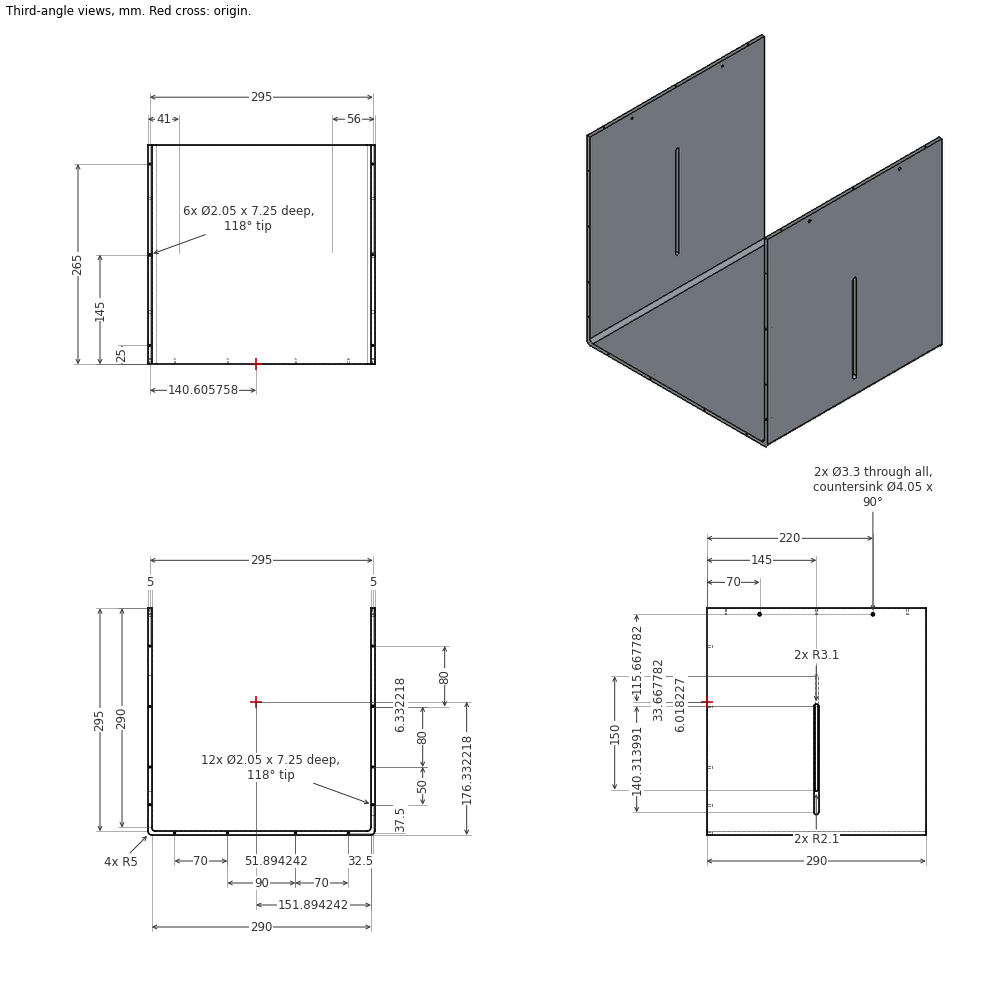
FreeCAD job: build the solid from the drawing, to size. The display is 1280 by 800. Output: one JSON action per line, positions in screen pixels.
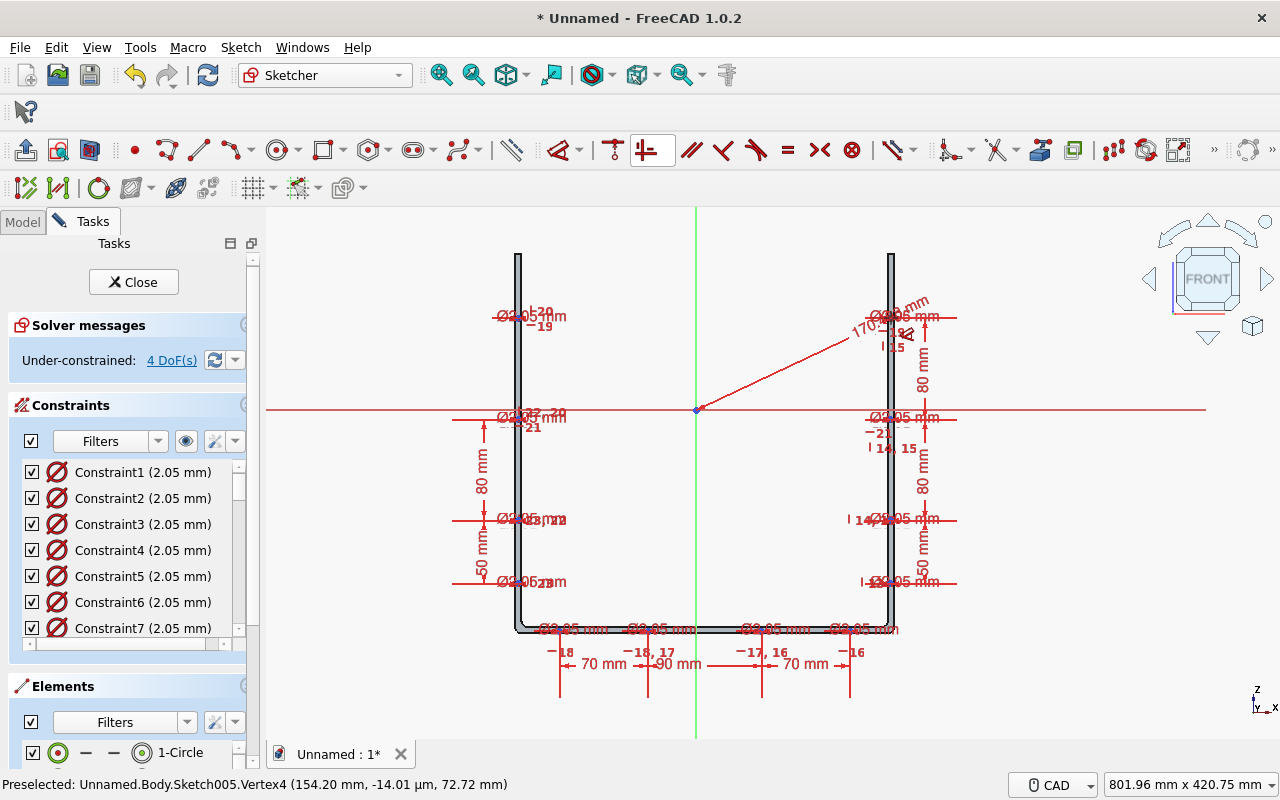
{"action": "left_click", "coordinate": [518, 318]}
{"action": "left_click", "coordinate": [619, 284]}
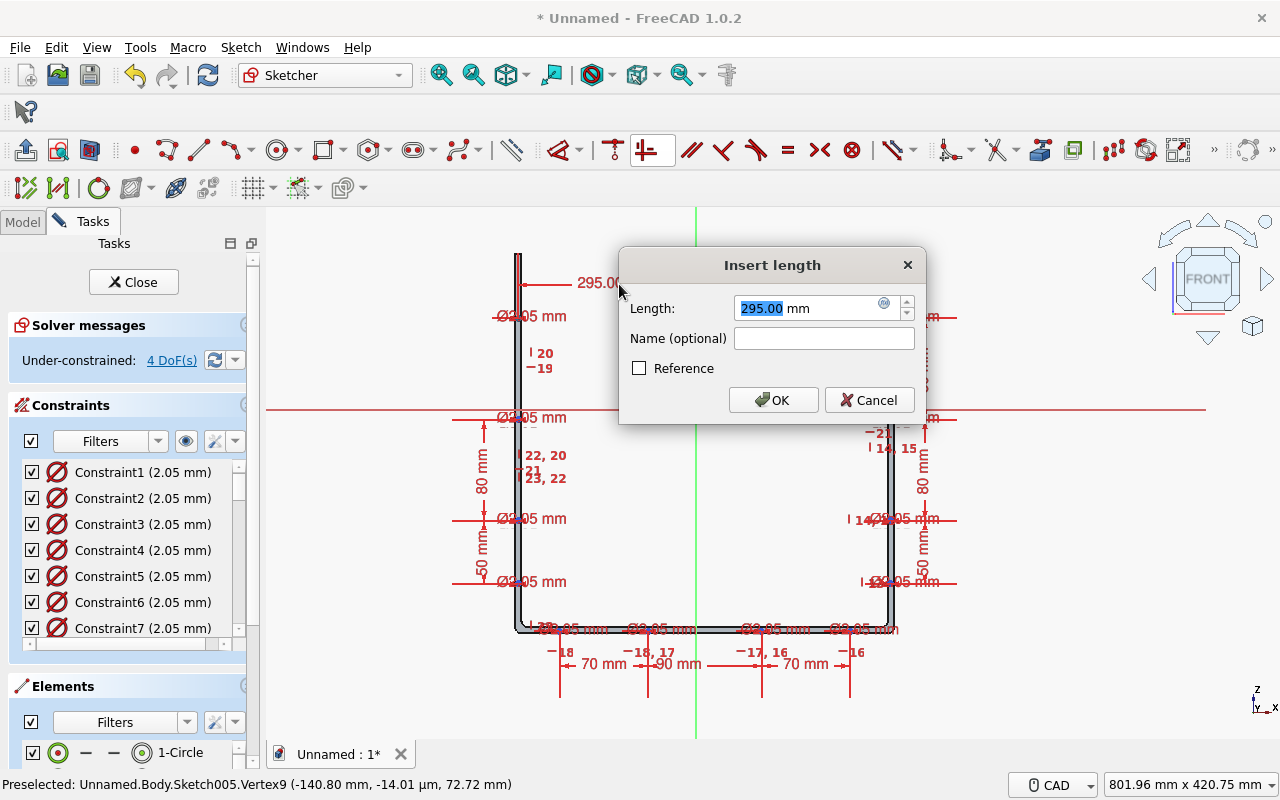
{"action": "type", "text": "295"}
{"action": "key", "text": "Return"}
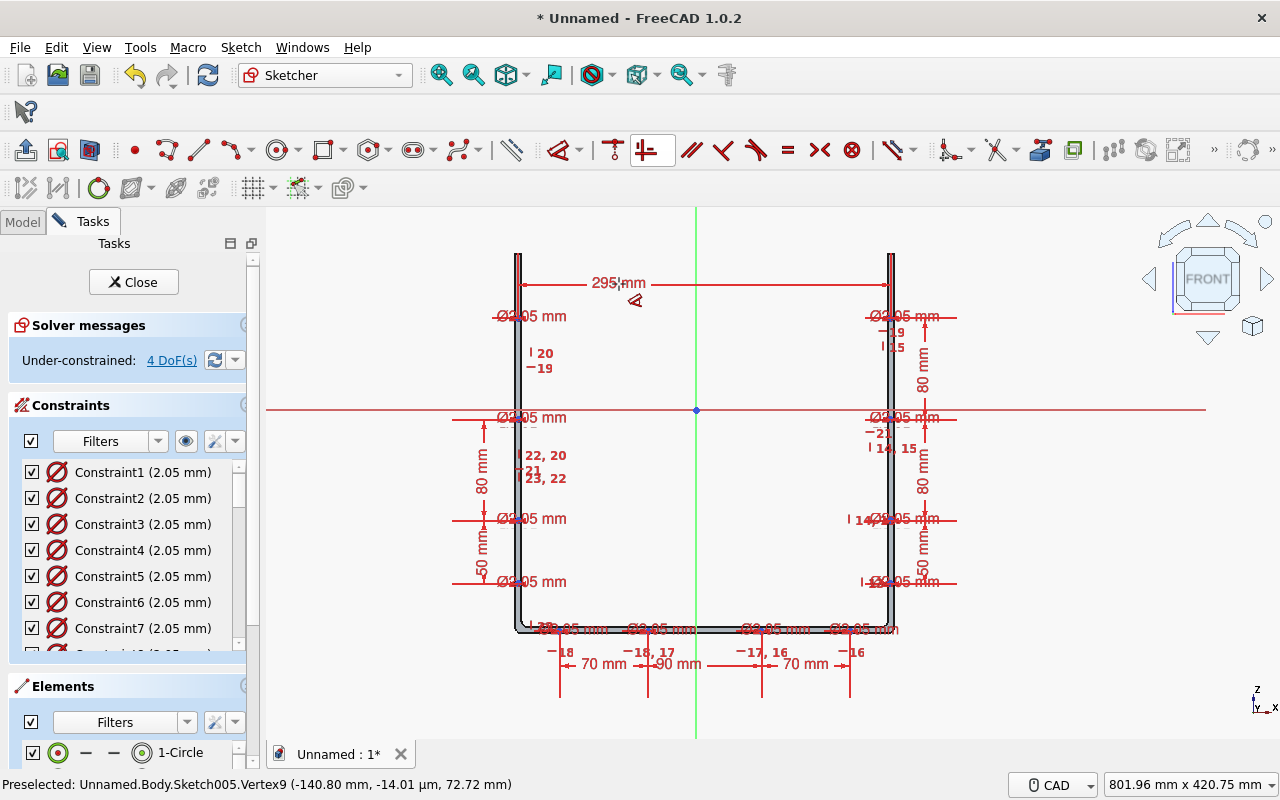
{"action": "left_click", "coordinate": [891, 584]}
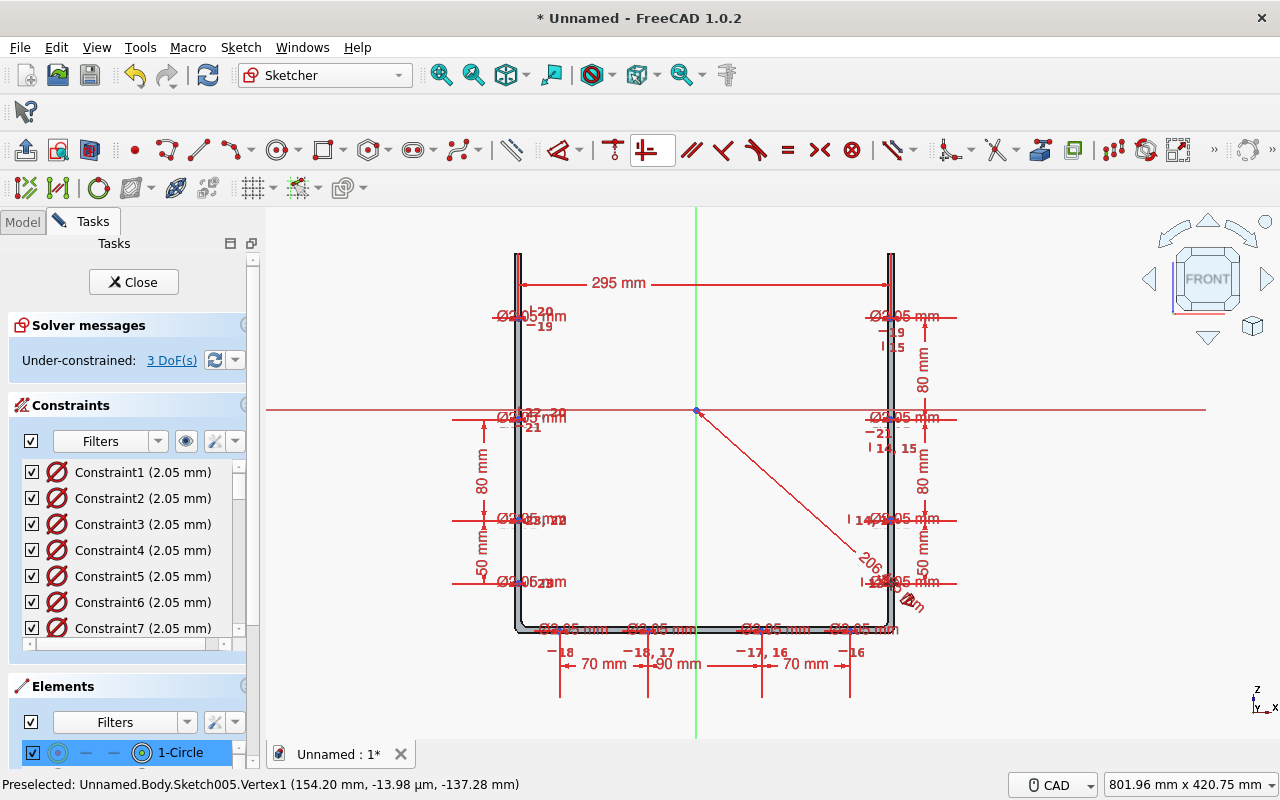
{"action": "left_click", "coordinate": [850, 631]}
{"action": "left_click", "coordinate": [880, 665]}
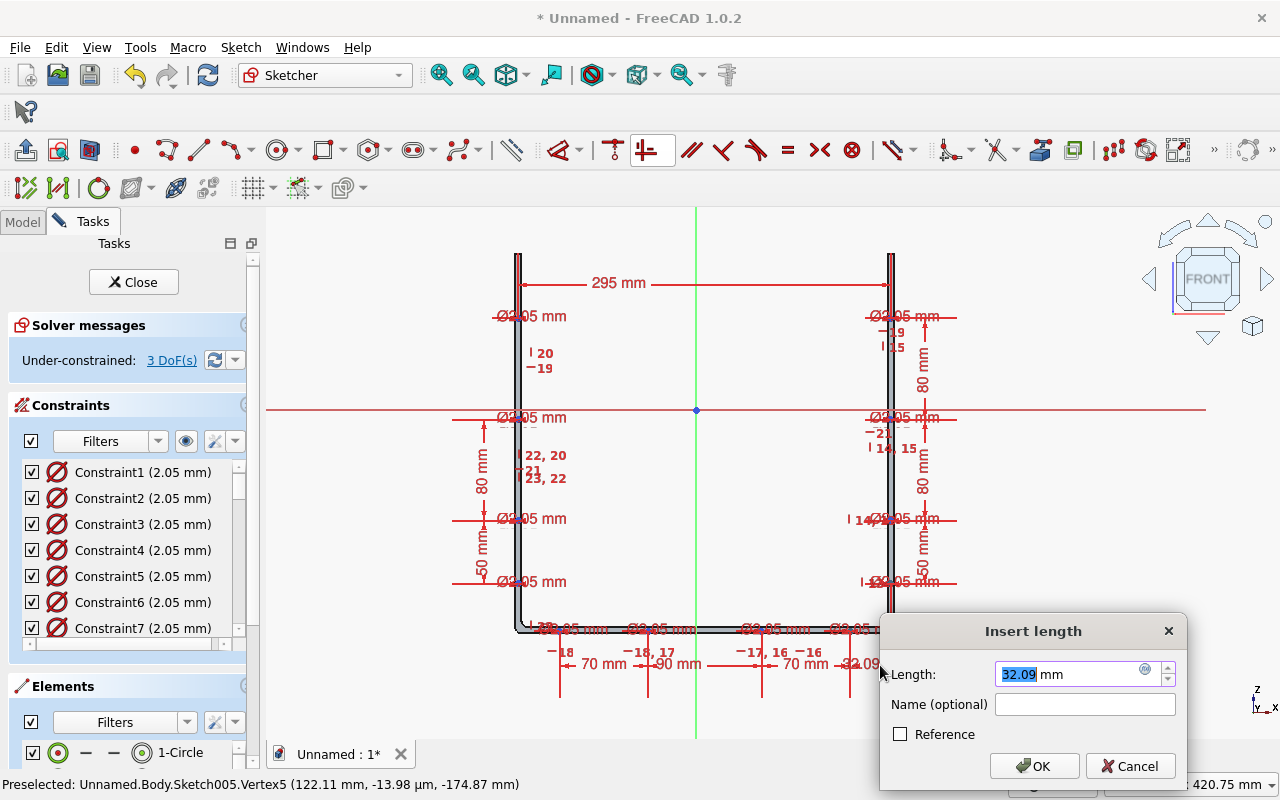
{"action": "type", "text": "32.5"}
{"action": "key", "text": "Return"}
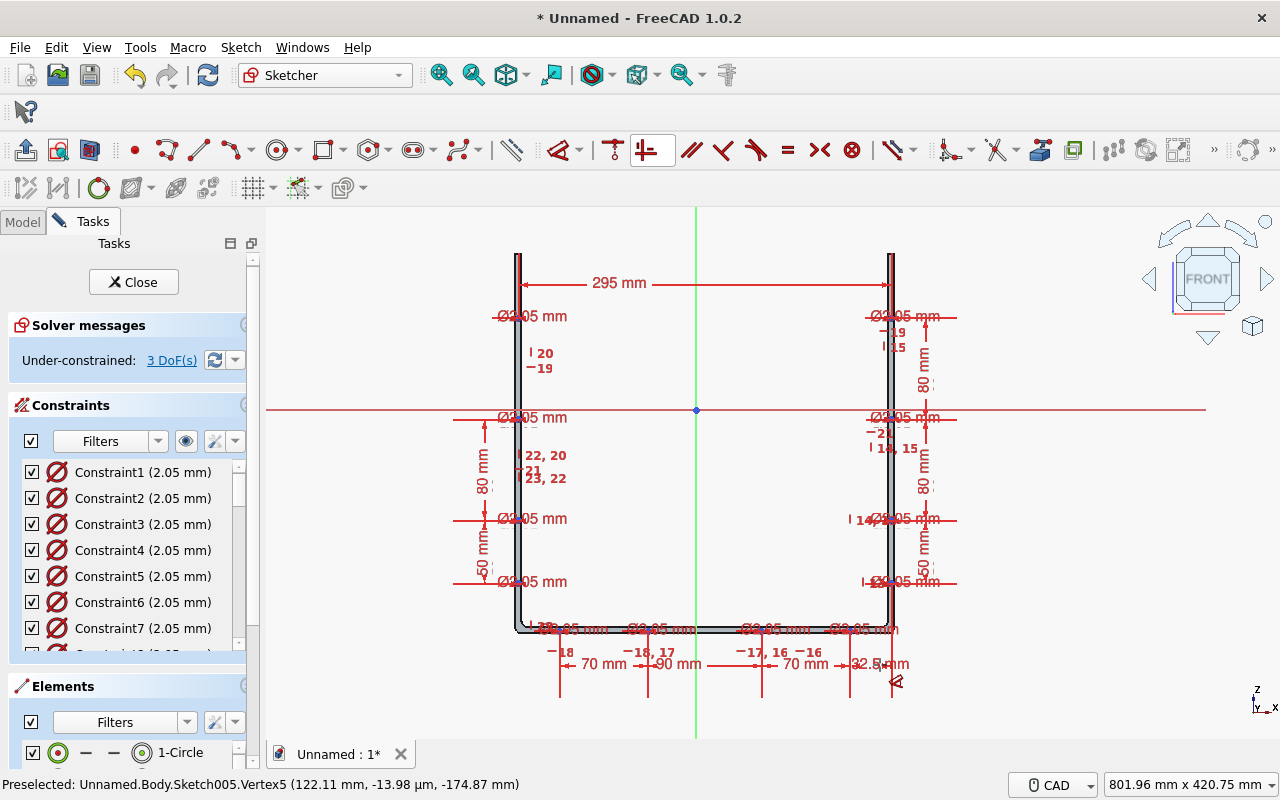
{"action": "left_click", "coordinate": [892, 584]}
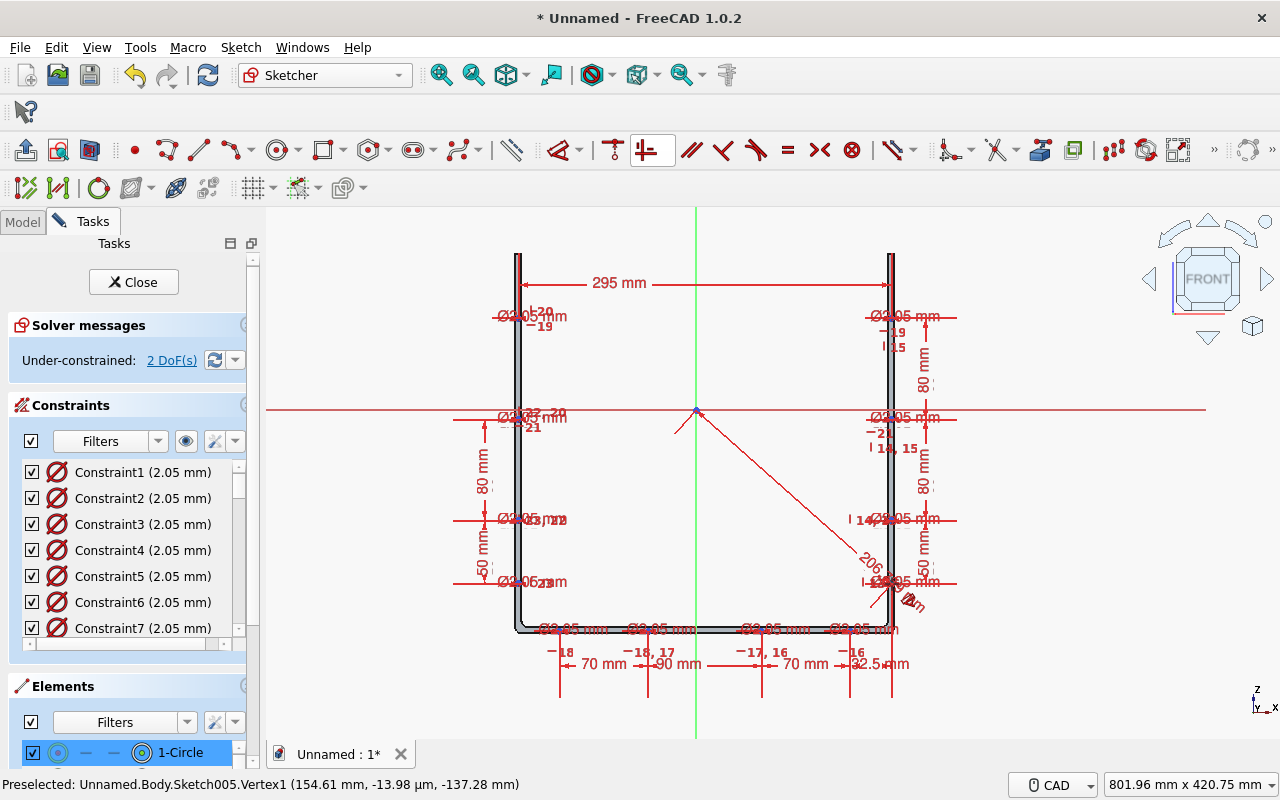
{"action": "left_click", "coordinate": [850, 631]}
{"action": "left_click", "coordinate": [926, 608]}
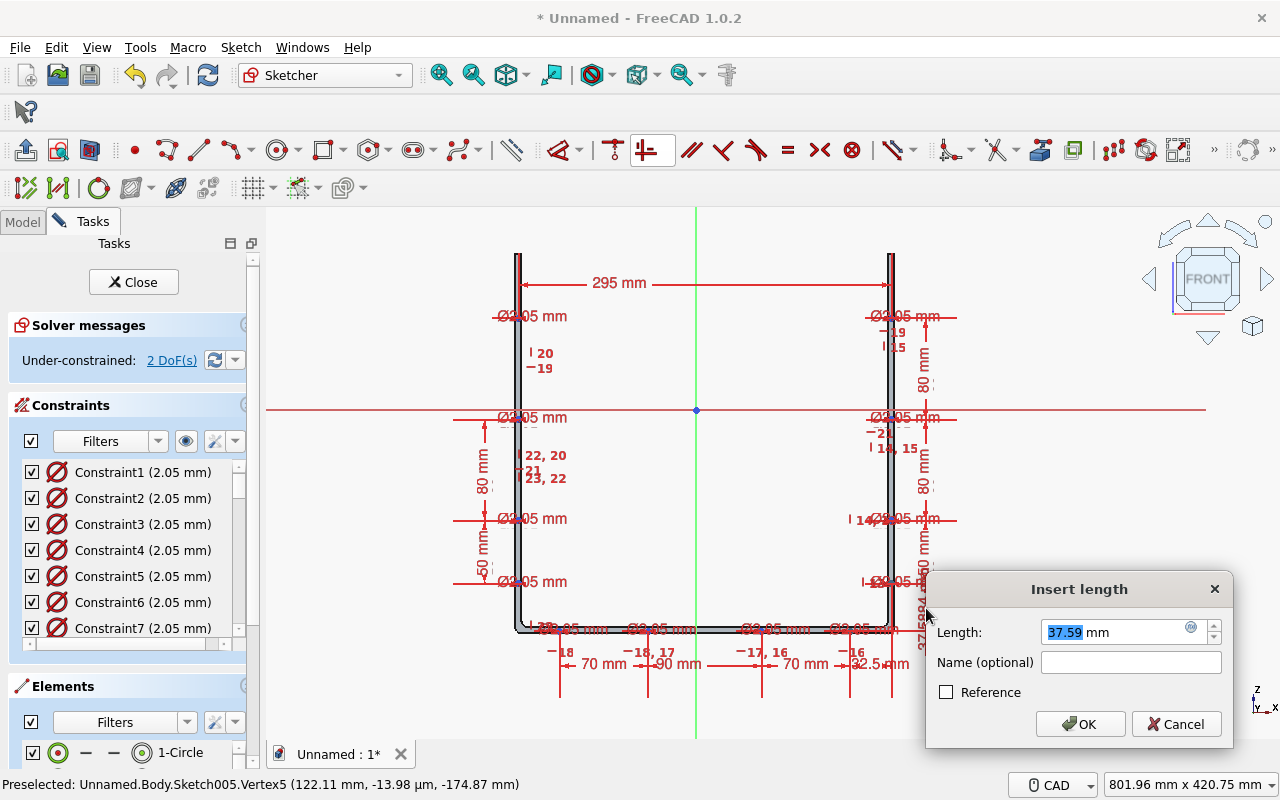
{"action": "type", "text": "37.5"}
{"action": "key", "text": "Return"}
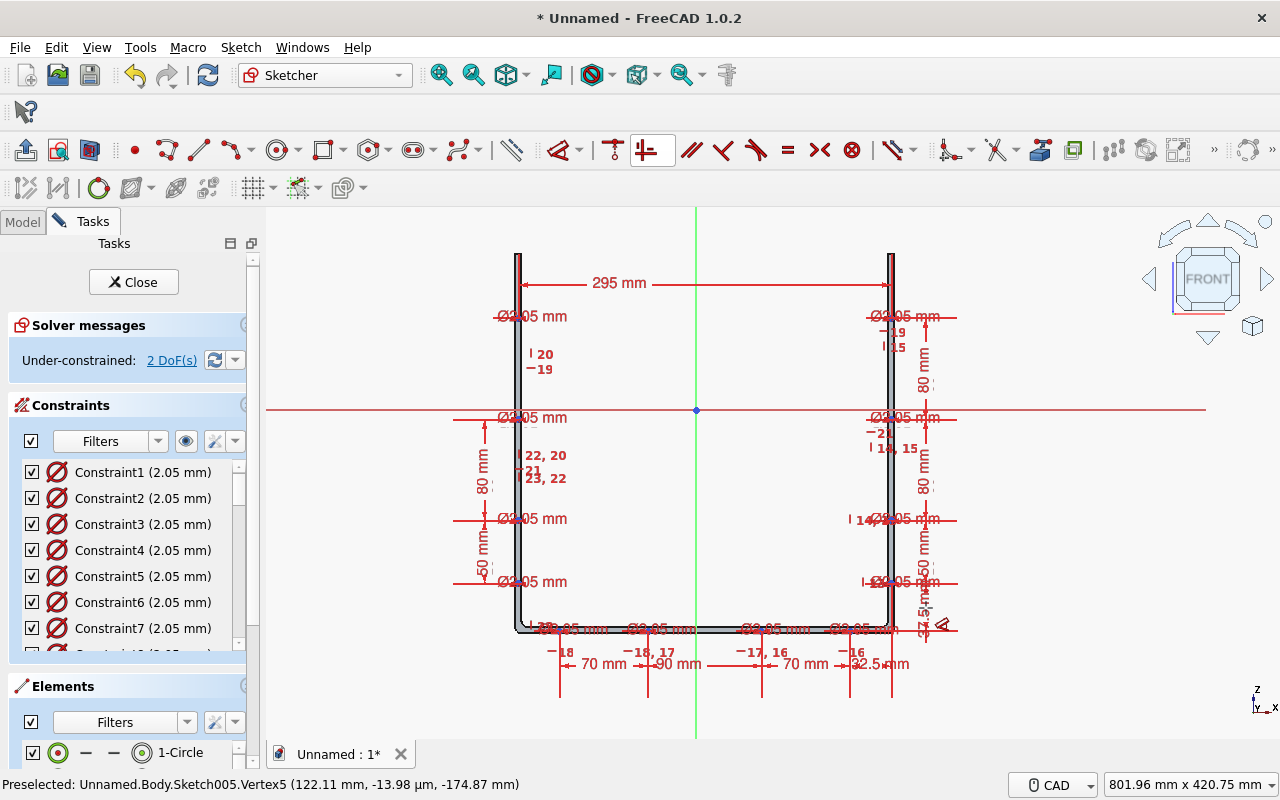
{"action": "scroll", "coordinate": [892, 420], "scroll_direction": "up", "scroll_amount": 9}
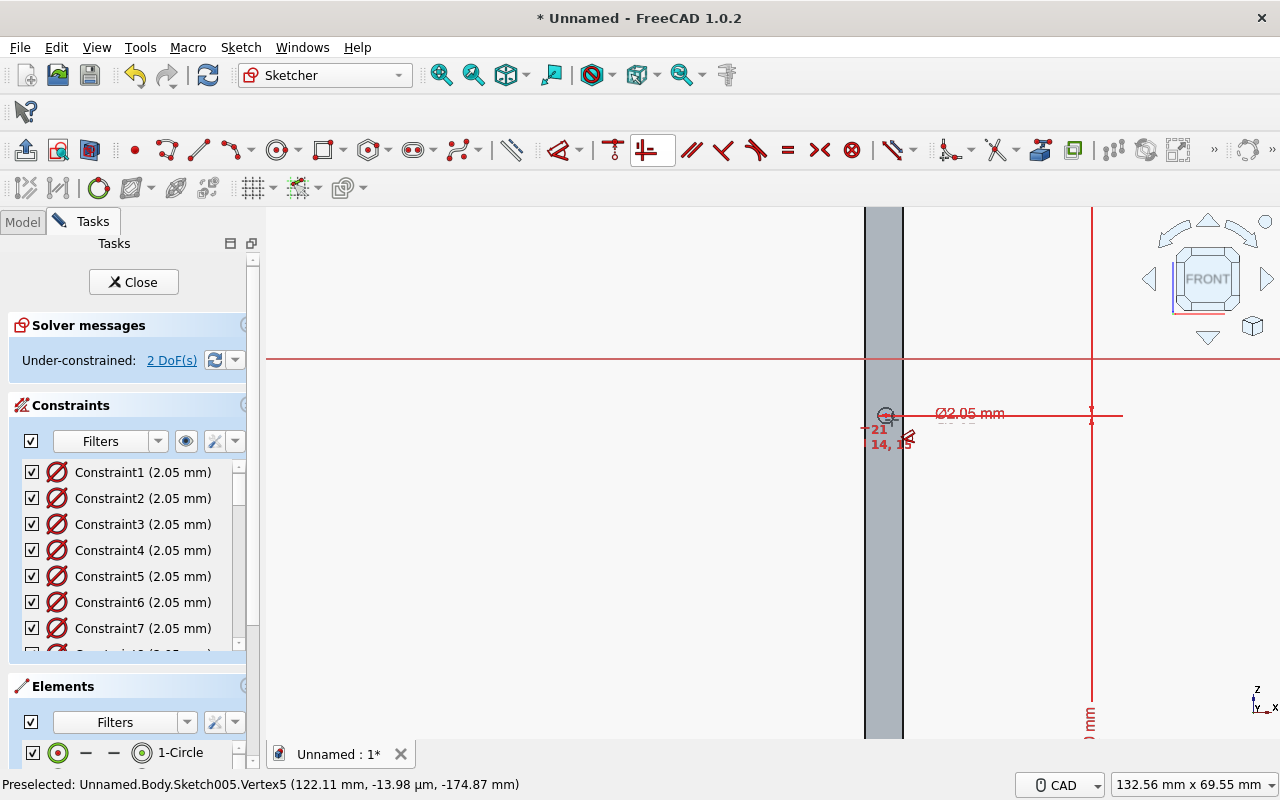
{"action": "left_click", "coordinate": [886, 416]}
{"action": "left_click", "coordinate": [920, 388]}